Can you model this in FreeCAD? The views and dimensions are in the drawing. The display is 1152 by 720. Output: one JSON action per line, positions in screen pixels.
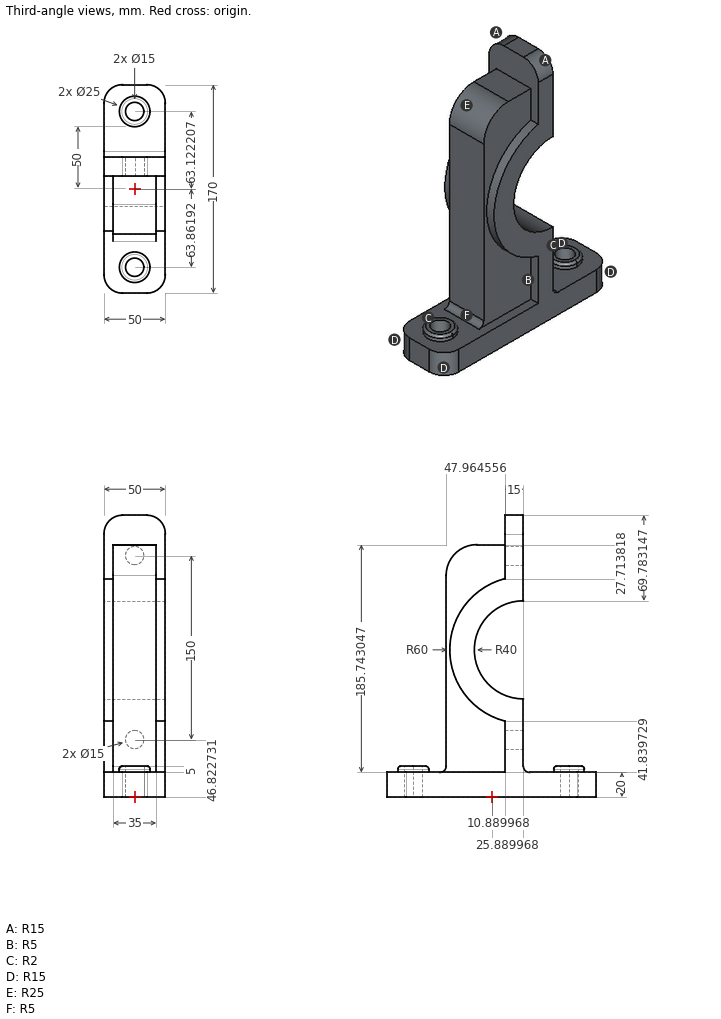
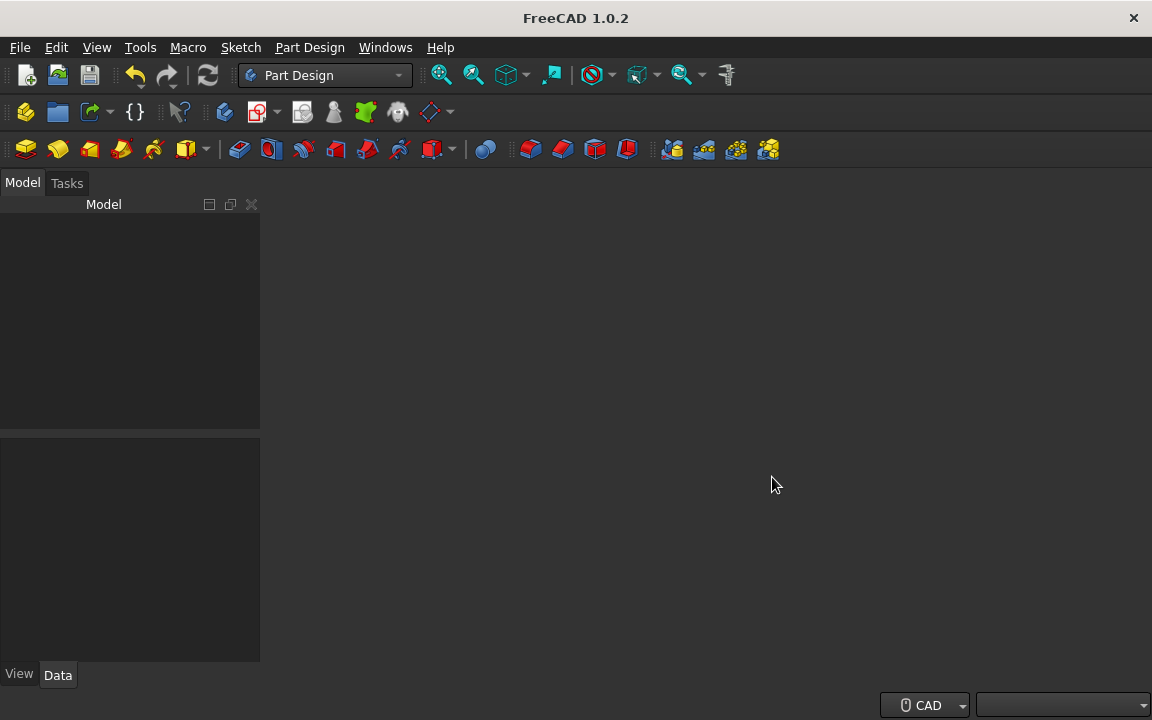
{"action": "left_click", "coordinate": [26, 76]}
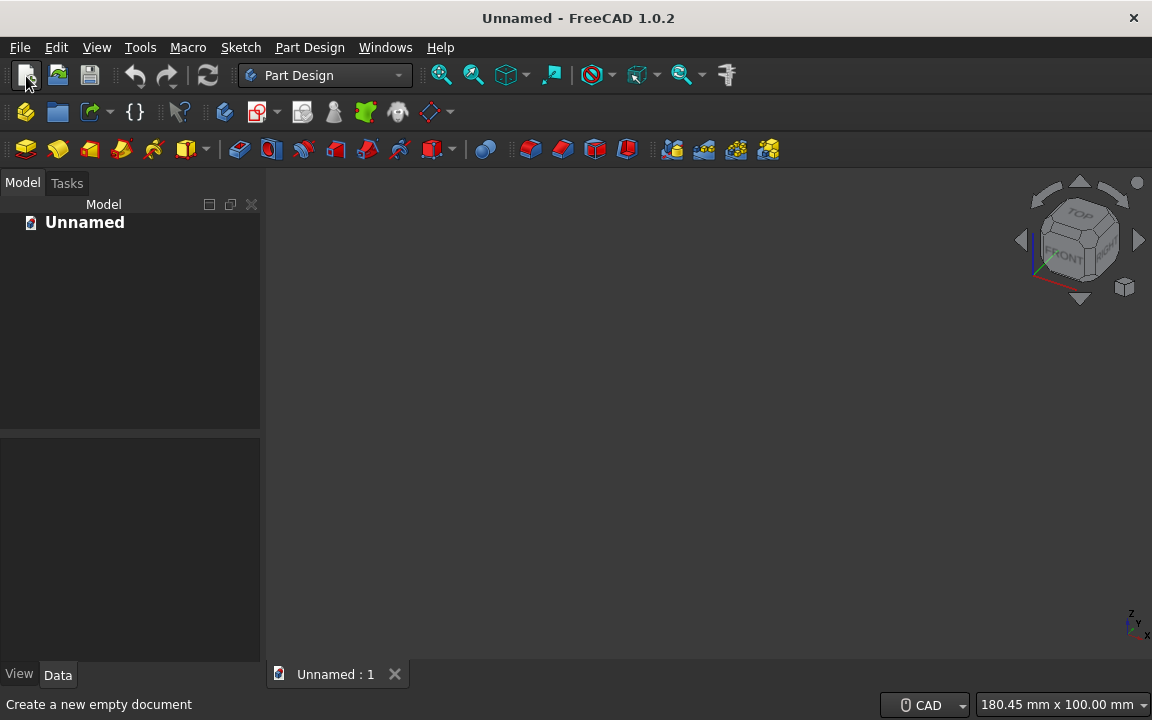
{"action": "left_click", "coordinate": [258, 112]}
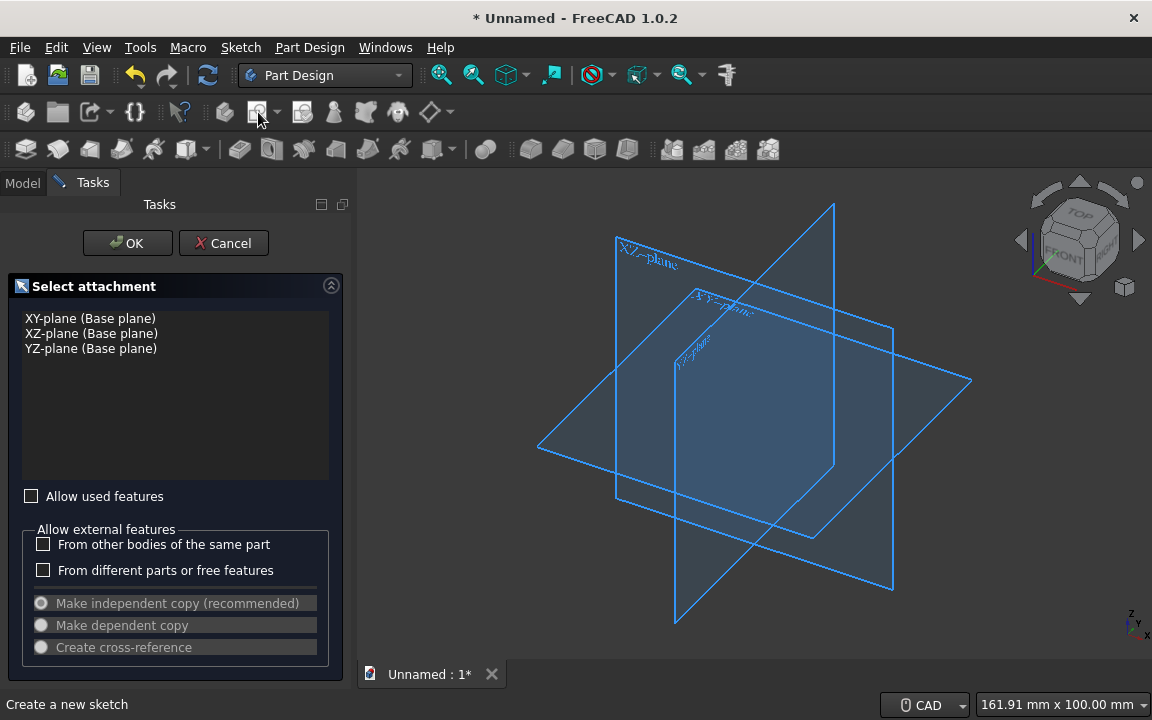
{"action": "left_click", "coordinate": [82, 318]}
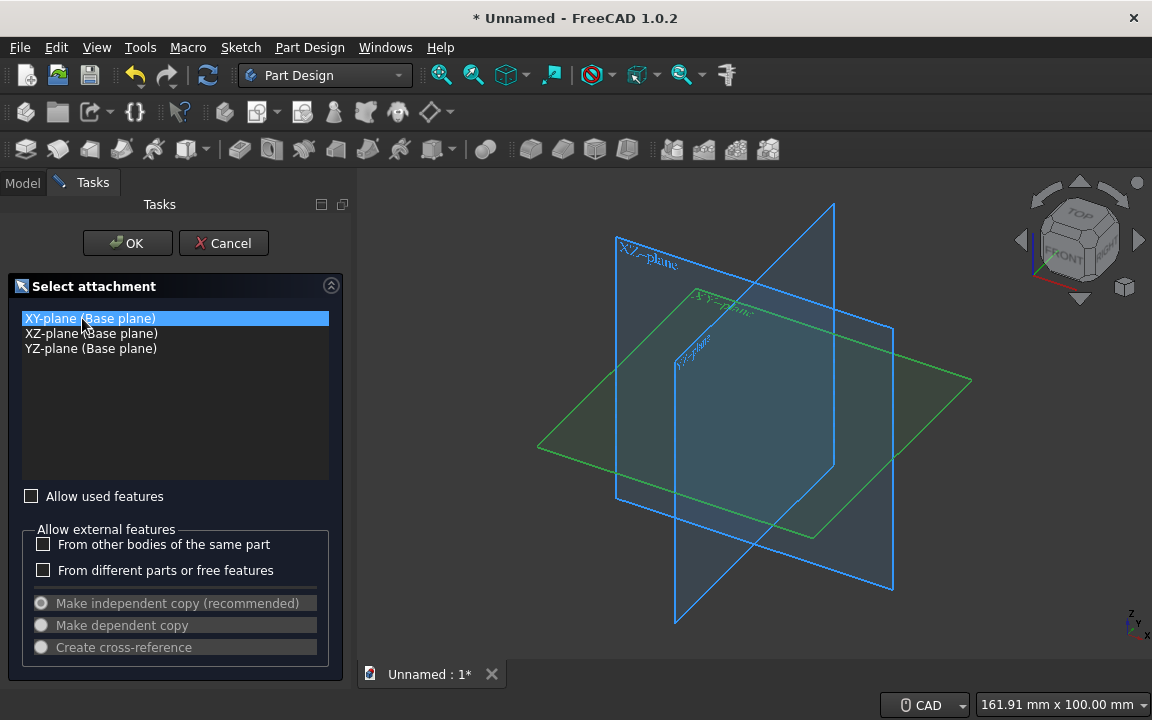
{"action": "left_click", "coordinate": [128, 243]}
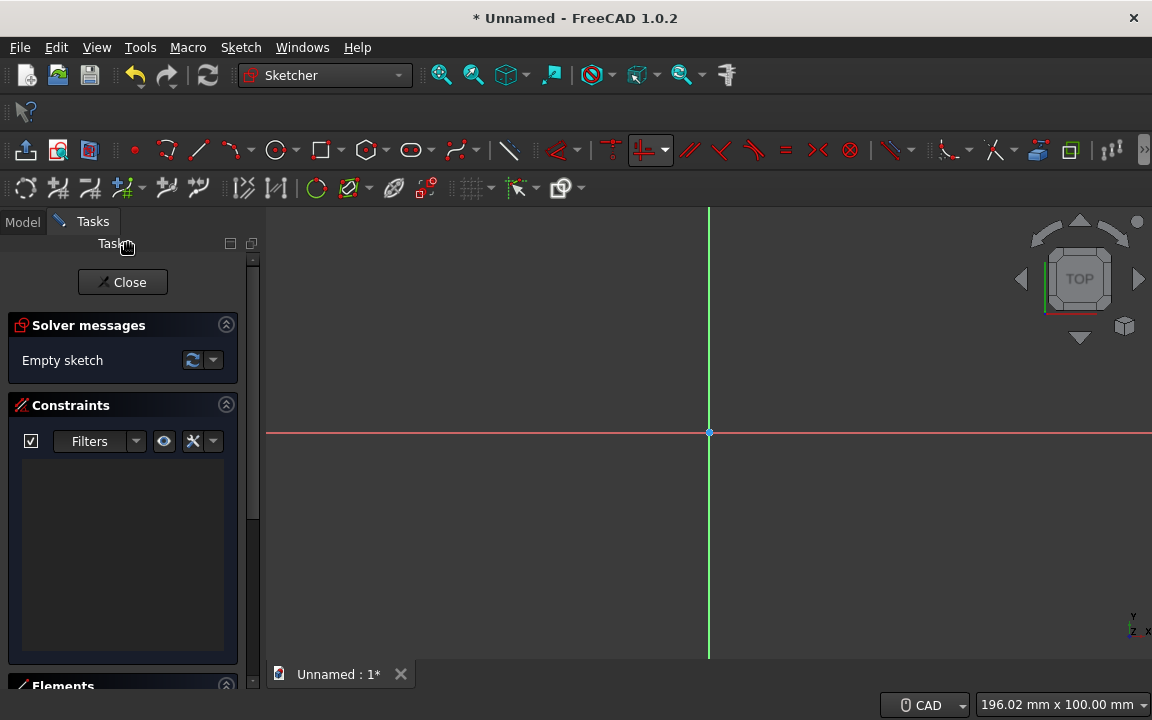
{"action": "scroll", "coordinate": [601, 433], "scroll_direction": "down", "scroll_amount": 5}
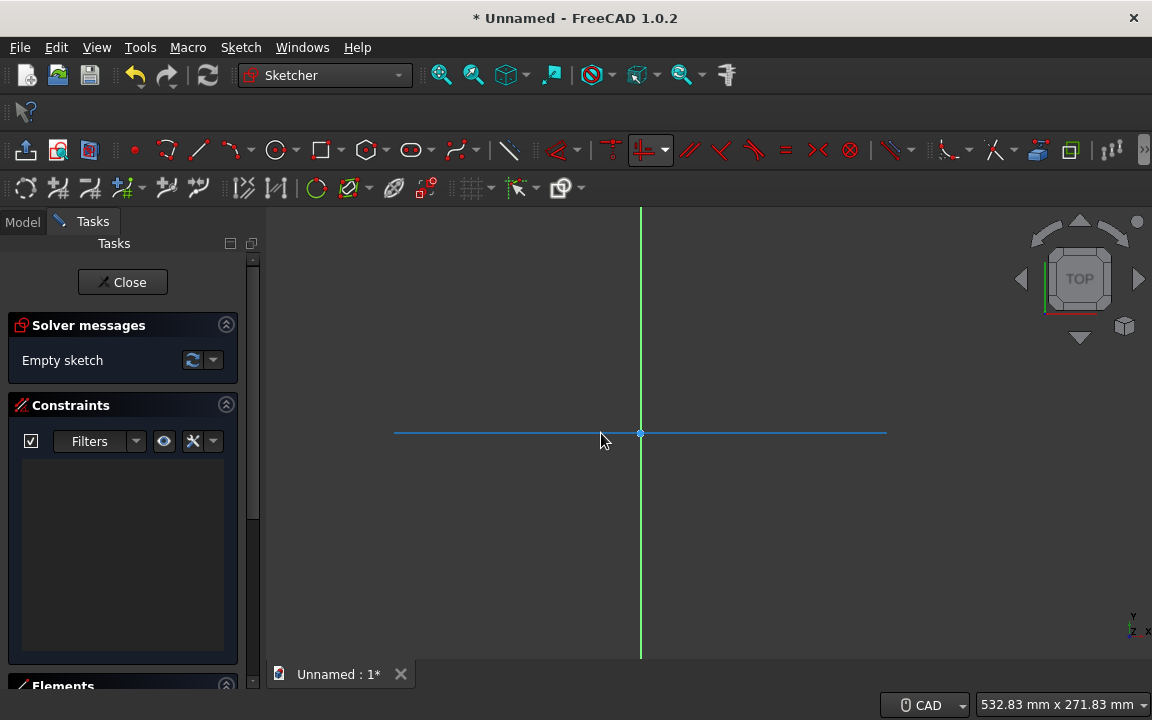
{"action": "key", "text": "g v"}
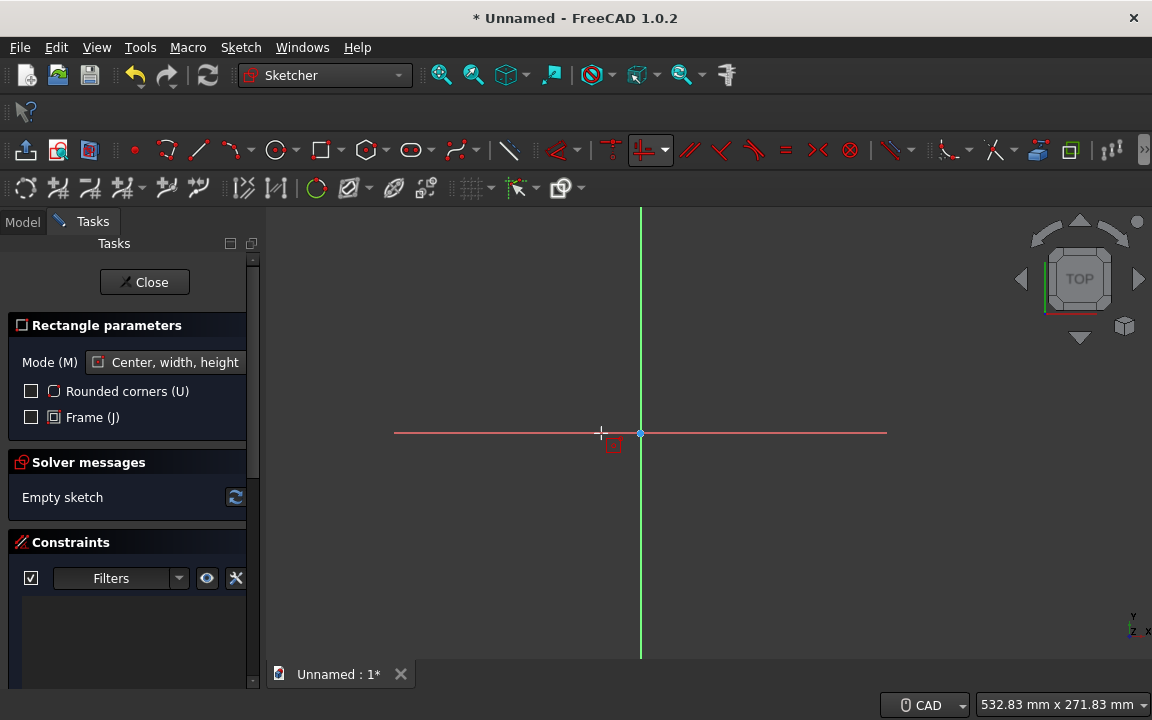
{"action": "left_click", "coordinate": [641, 433]}
{"action": "mouse_move", "coordinate": [683, 292]}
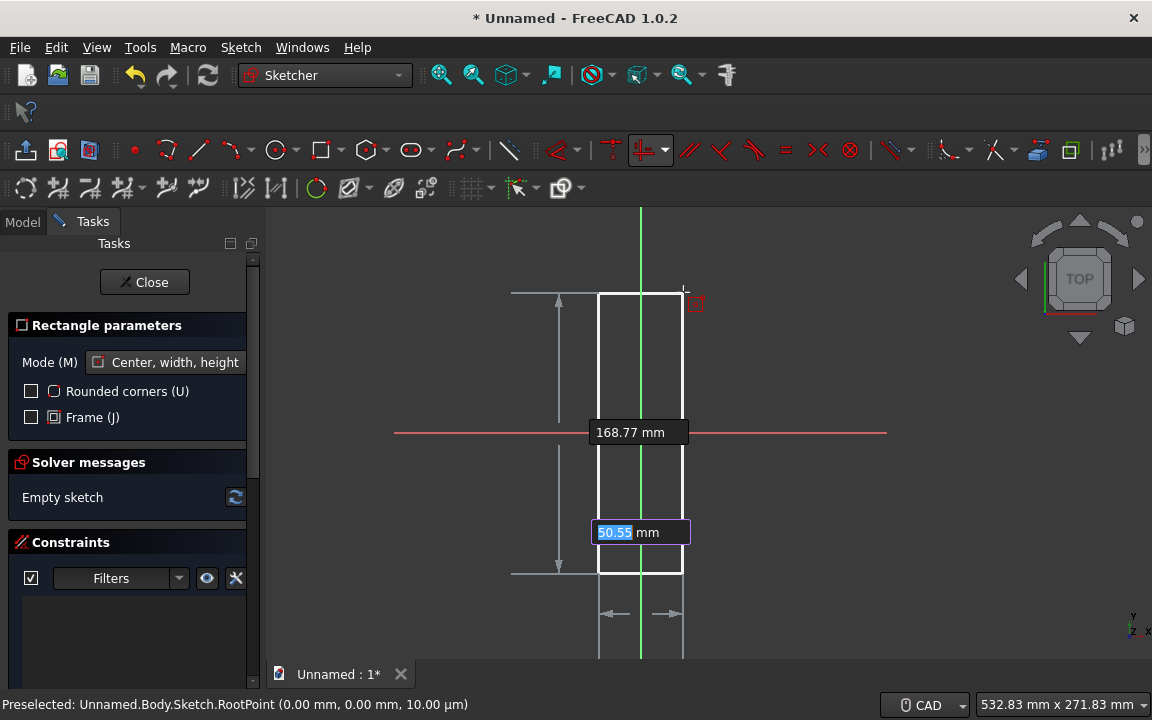
{"action": "type", "text": "50"}
{"action": "key", "text": "Tab"}
{"action": "type", "text": "170"}
{"action": "key", "text": "Return"}
{"action": "key", "text": "Escape"}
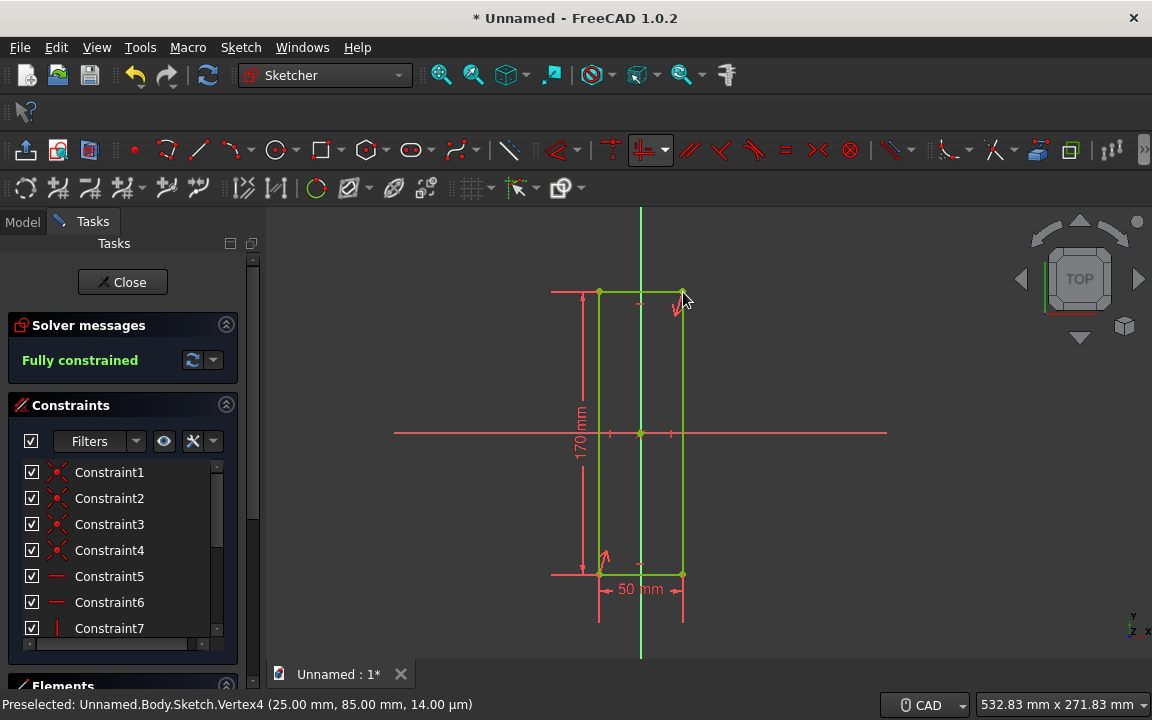
{"action": "left_click", "coordinate": [123, 282]}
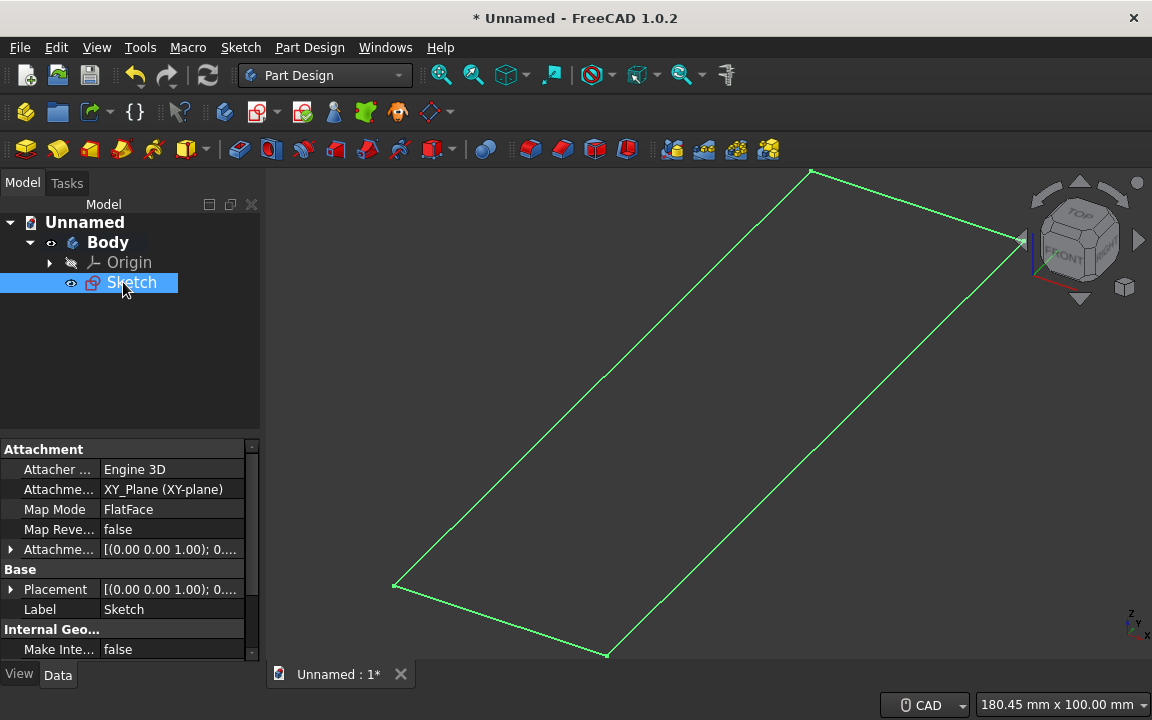
{"action": "left_click", "coordinate": [26, 150]}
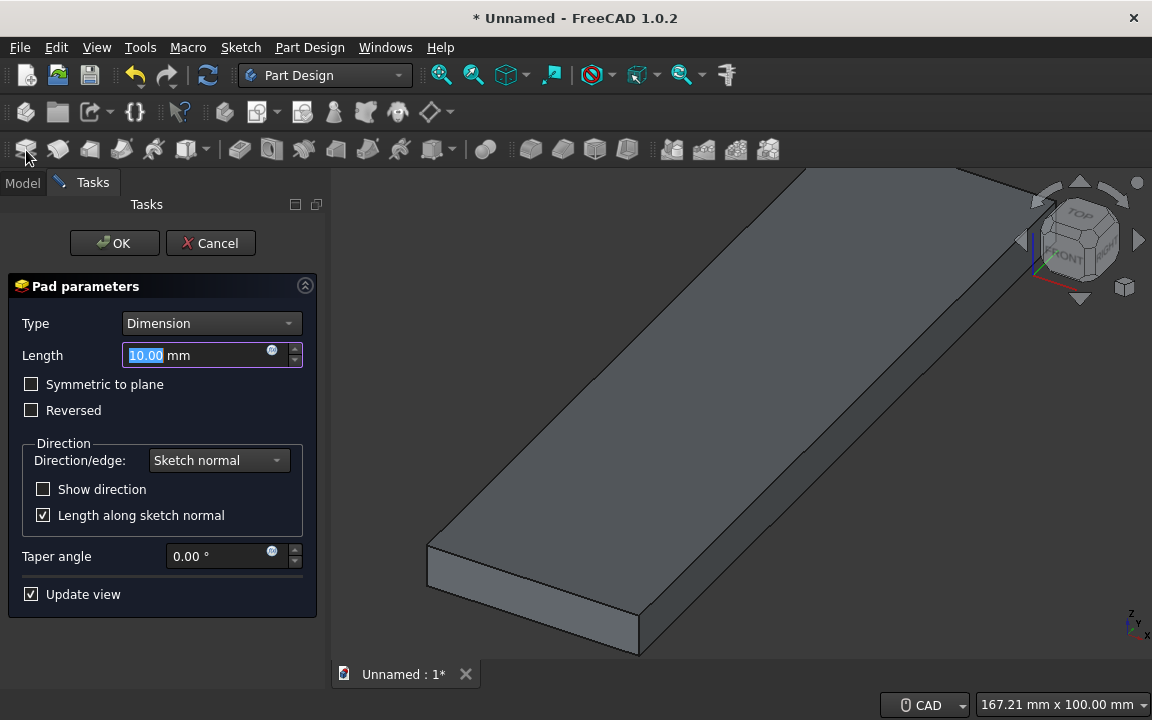
{"action": "type", "text": "20"}
{"action": "key", "text": "Tab"}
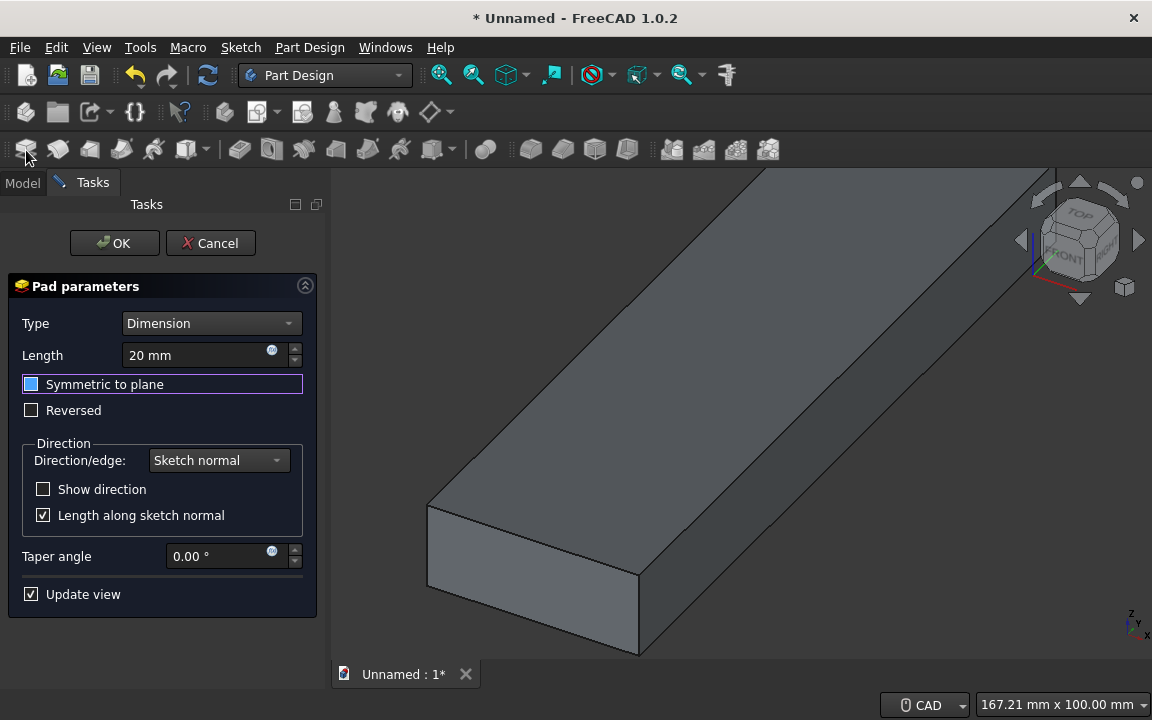
{"action": "left_click", "coordinate": [115, 243]}